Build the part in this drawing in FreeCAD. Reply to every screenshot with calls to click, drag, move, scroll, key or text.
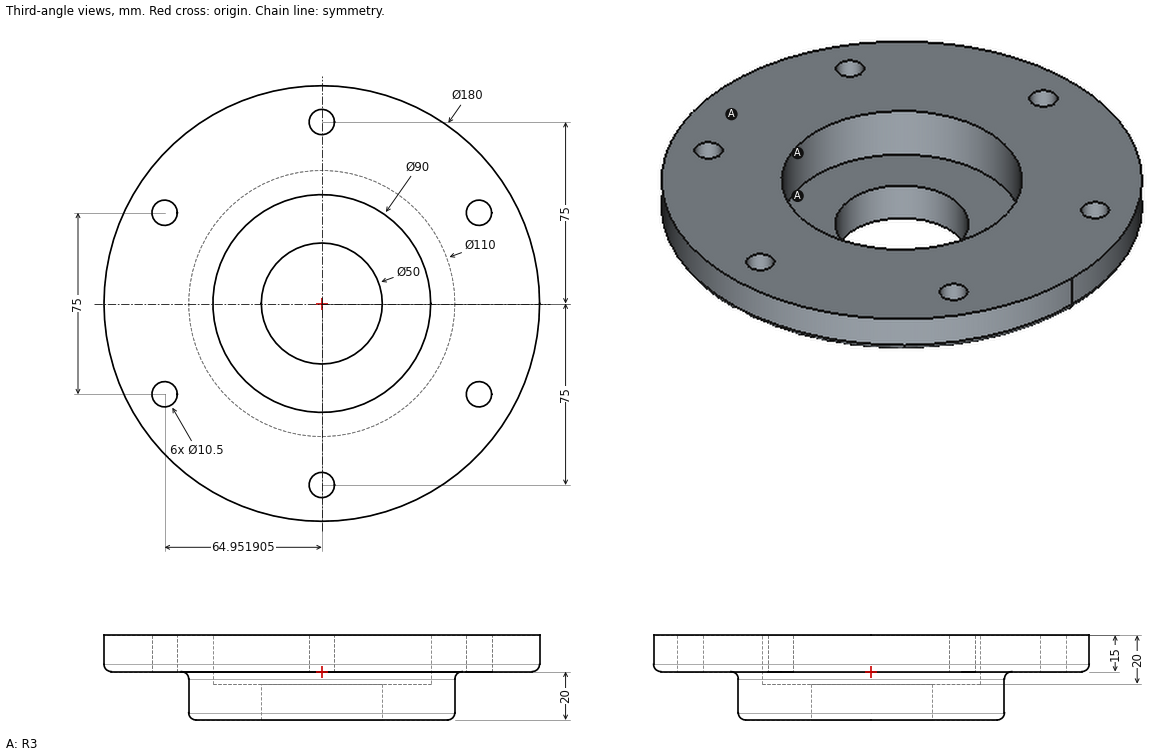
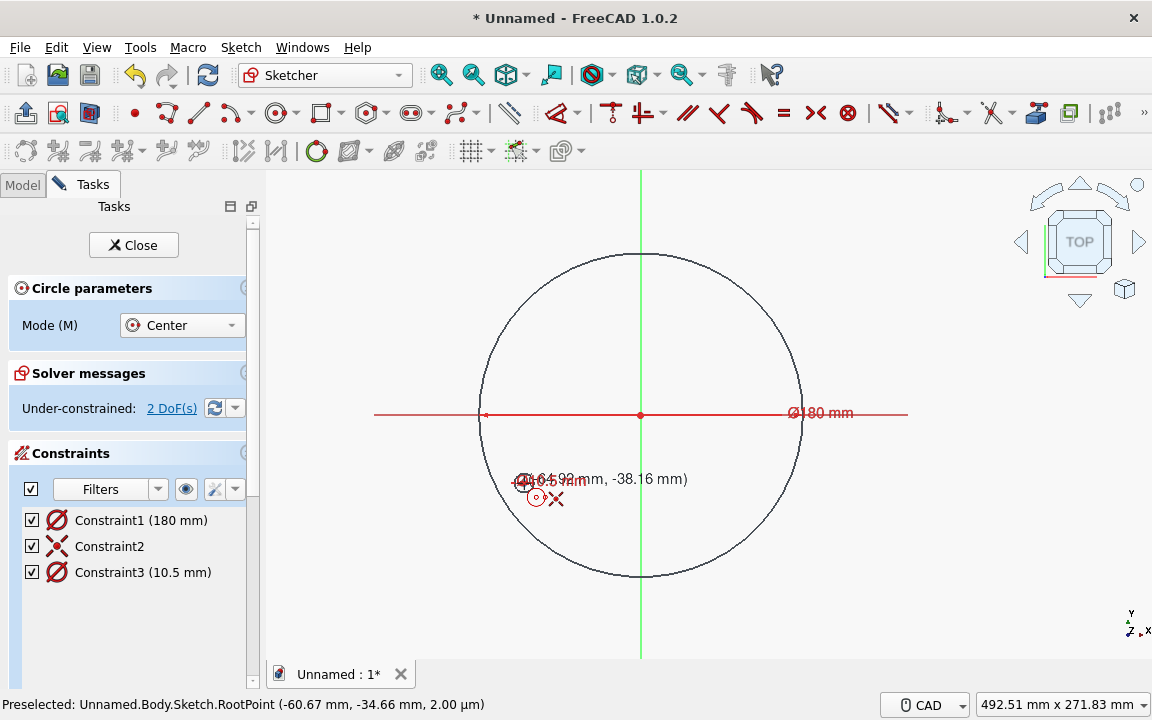
scroll(641, 550, up, 5)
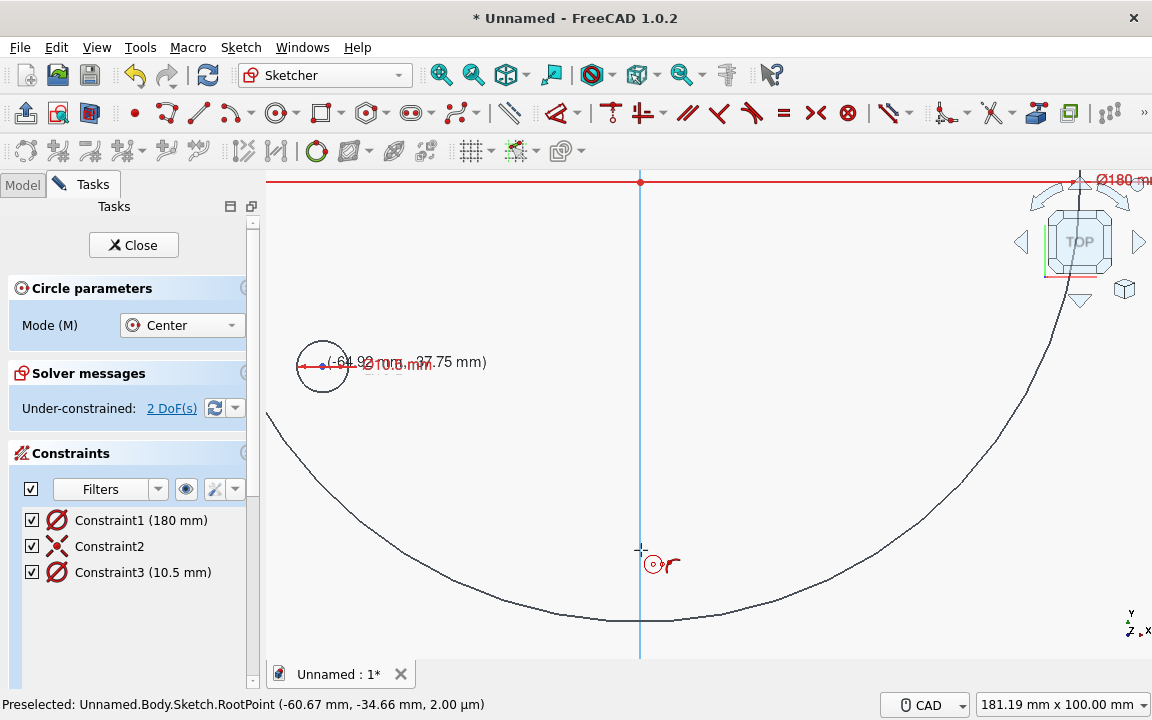
click(640, 549)
move(658, 531)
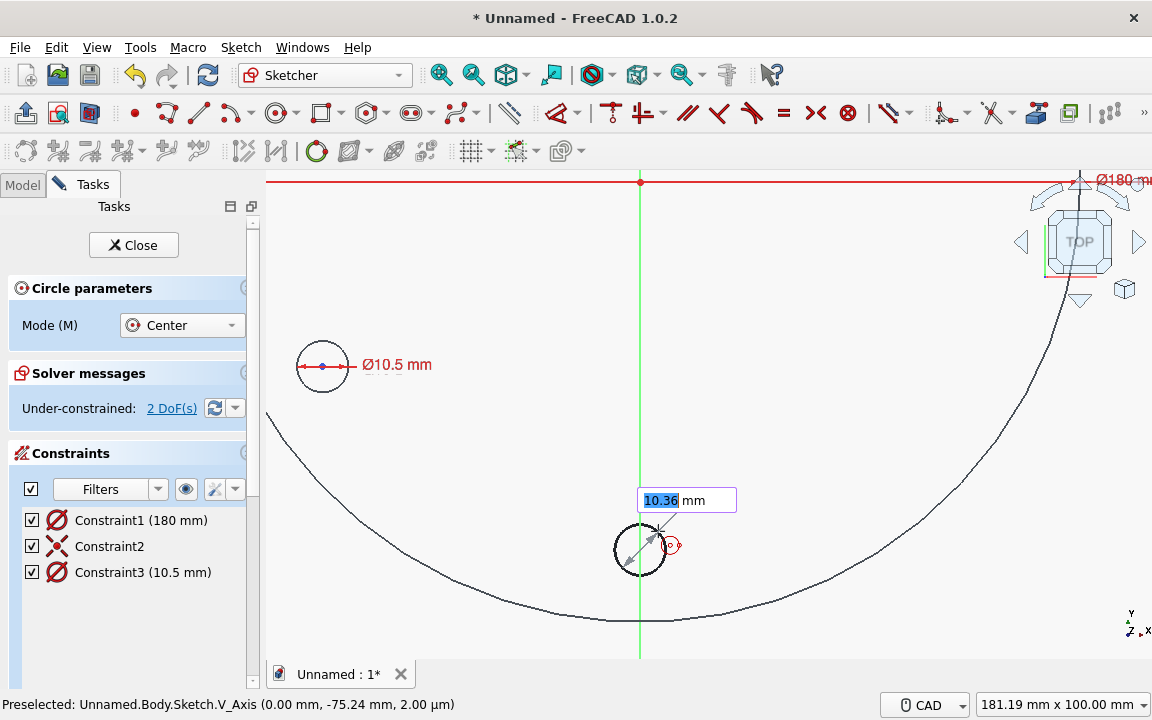
text(10.5)
key(Return)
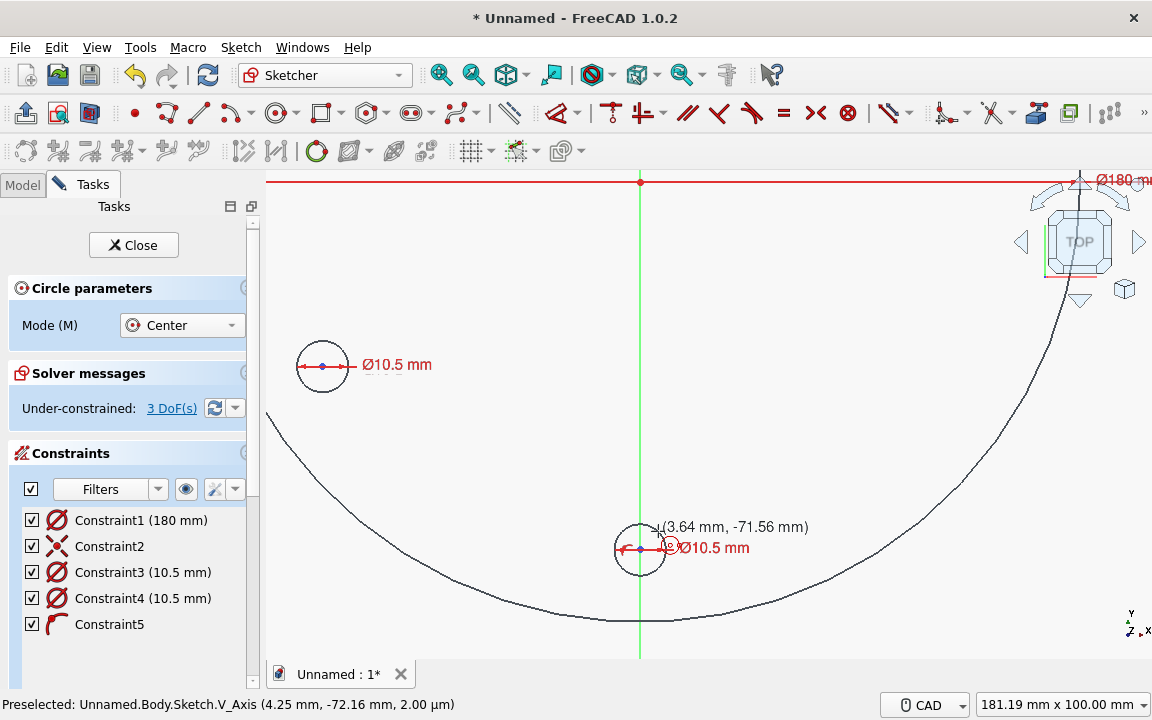
click(958, 365)
move(976, 347)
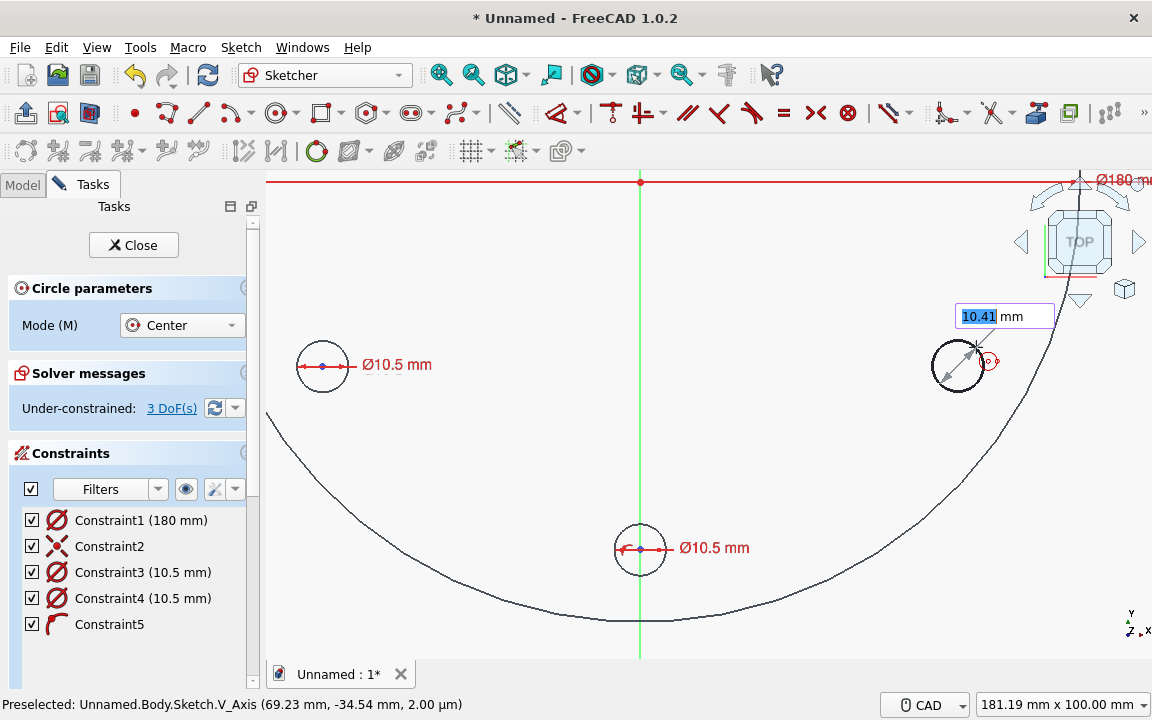
text(10.5)
key(Return)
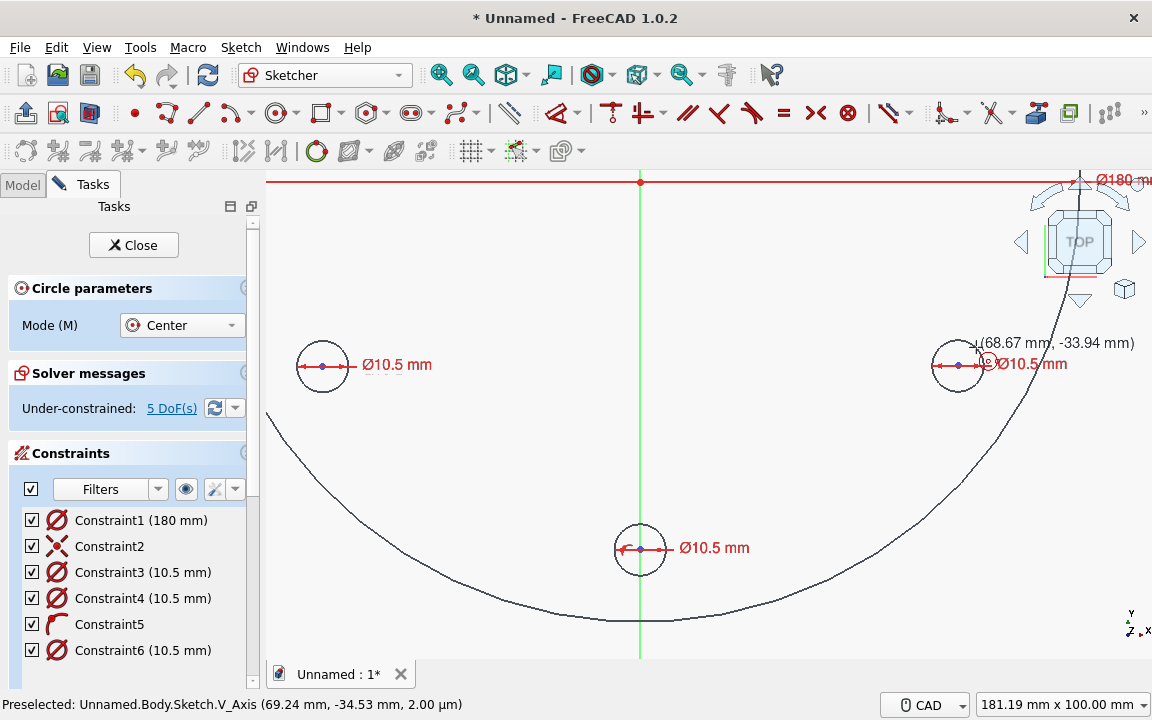
scroll(641, 550, down, 5)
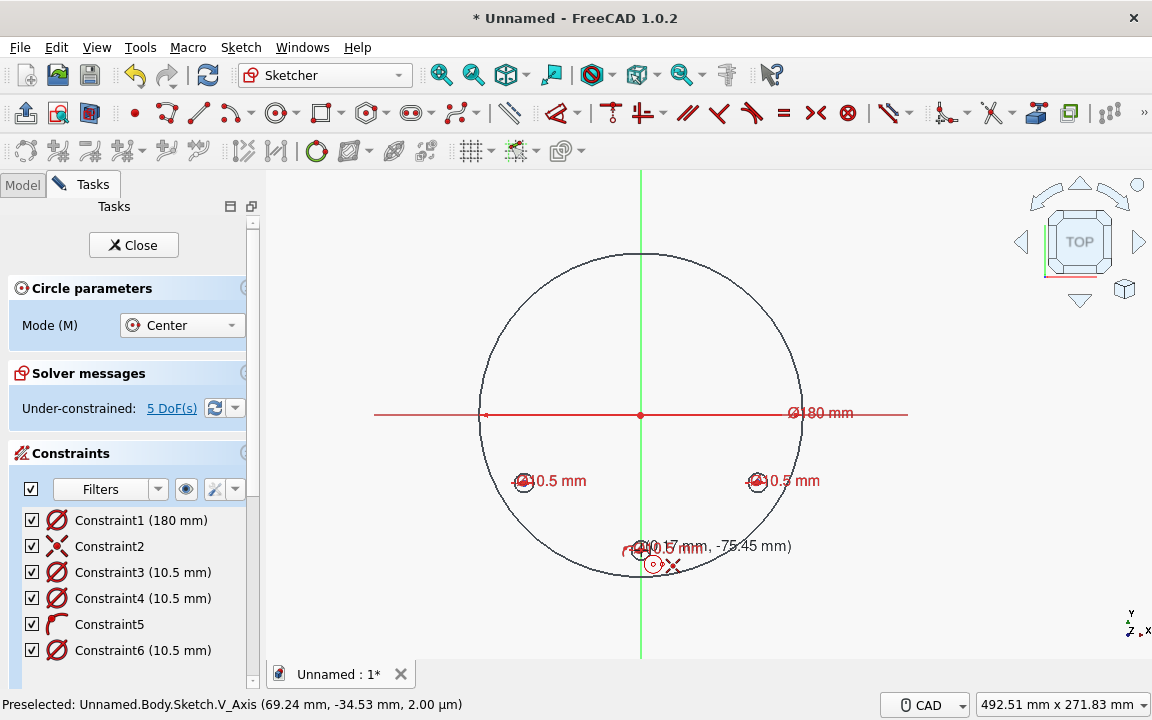
scroll(524, 348, up, 5)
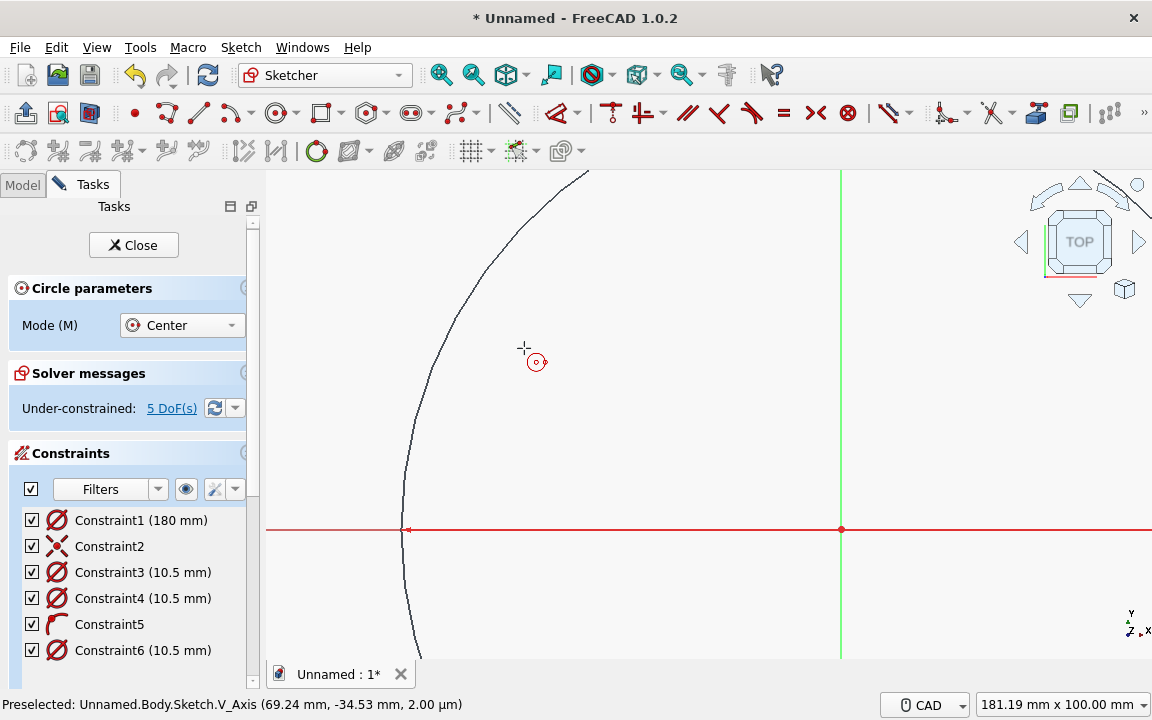
click(524, 346)
move(542, 328)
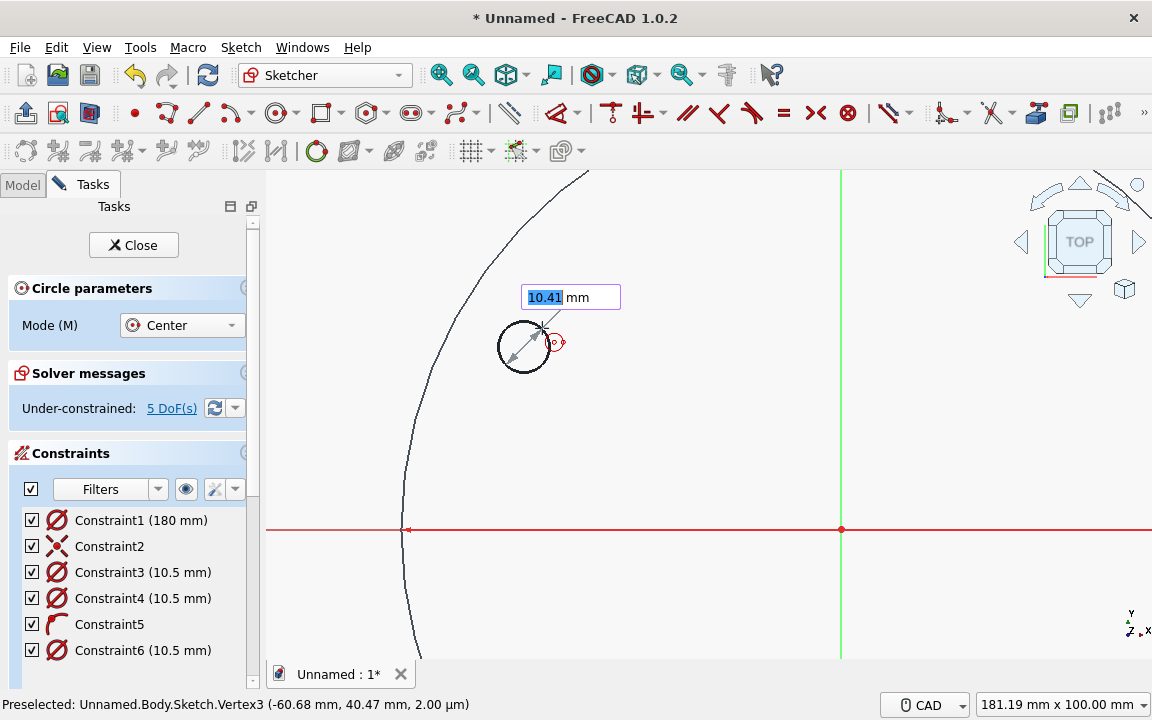
text(10.5)
key(Return)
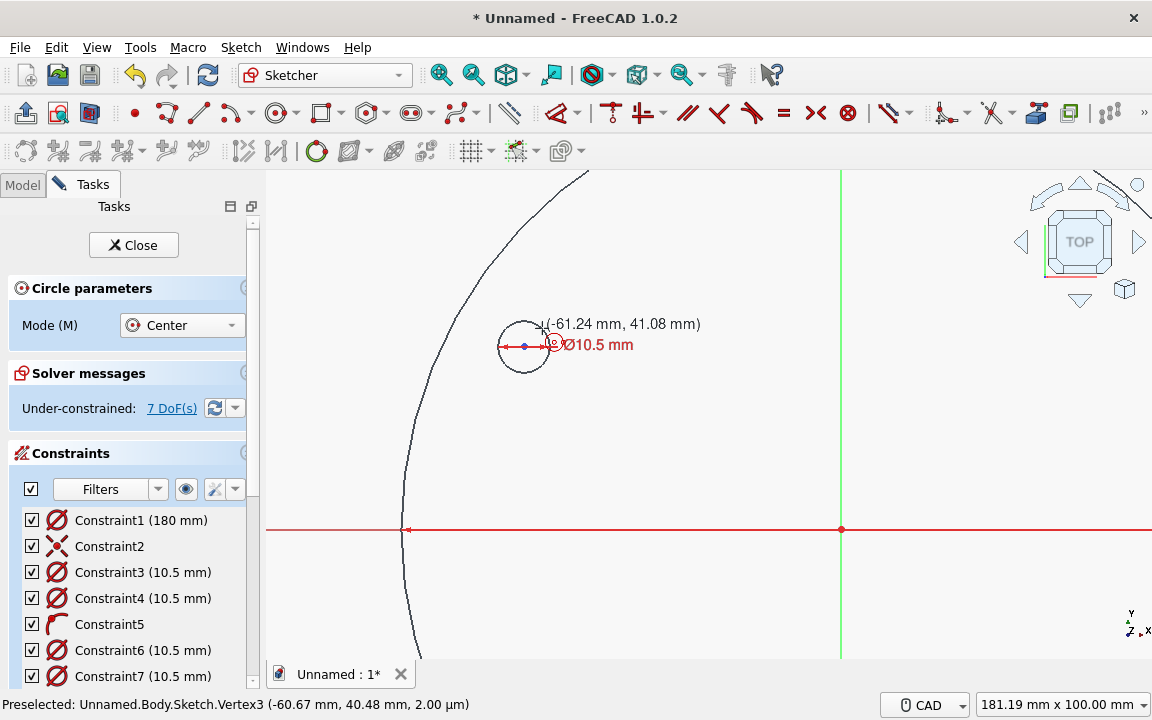
click(841, 530)
move(928, 443)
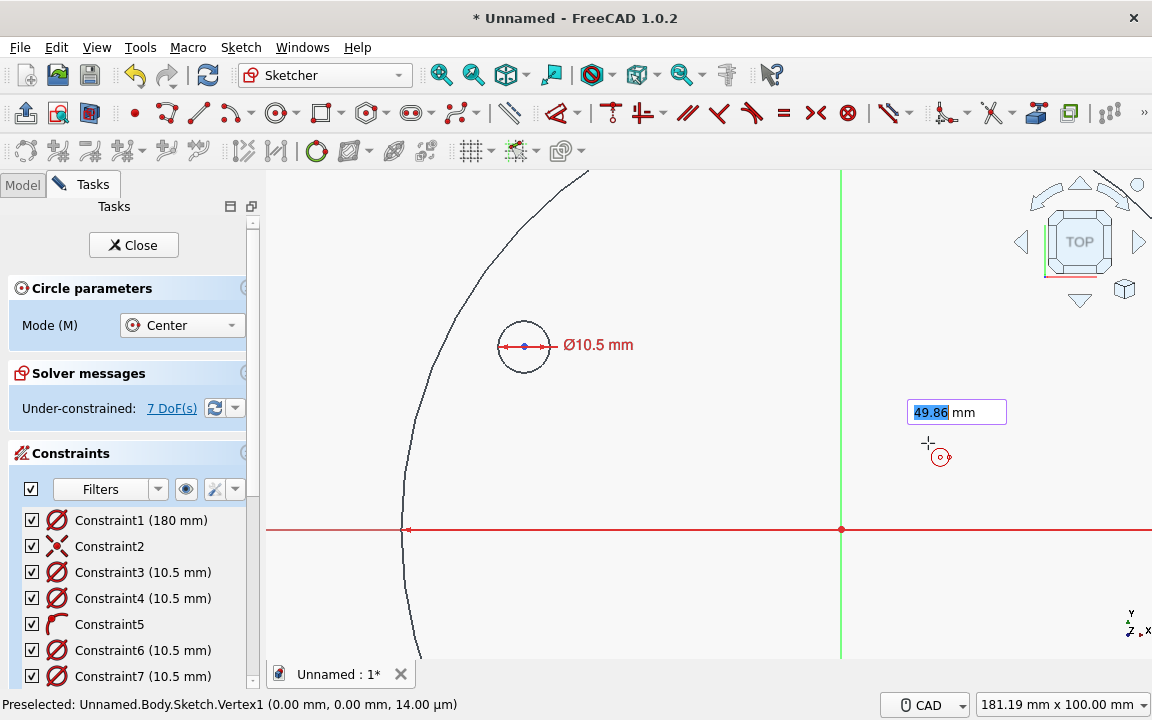
text(50)
key(Return)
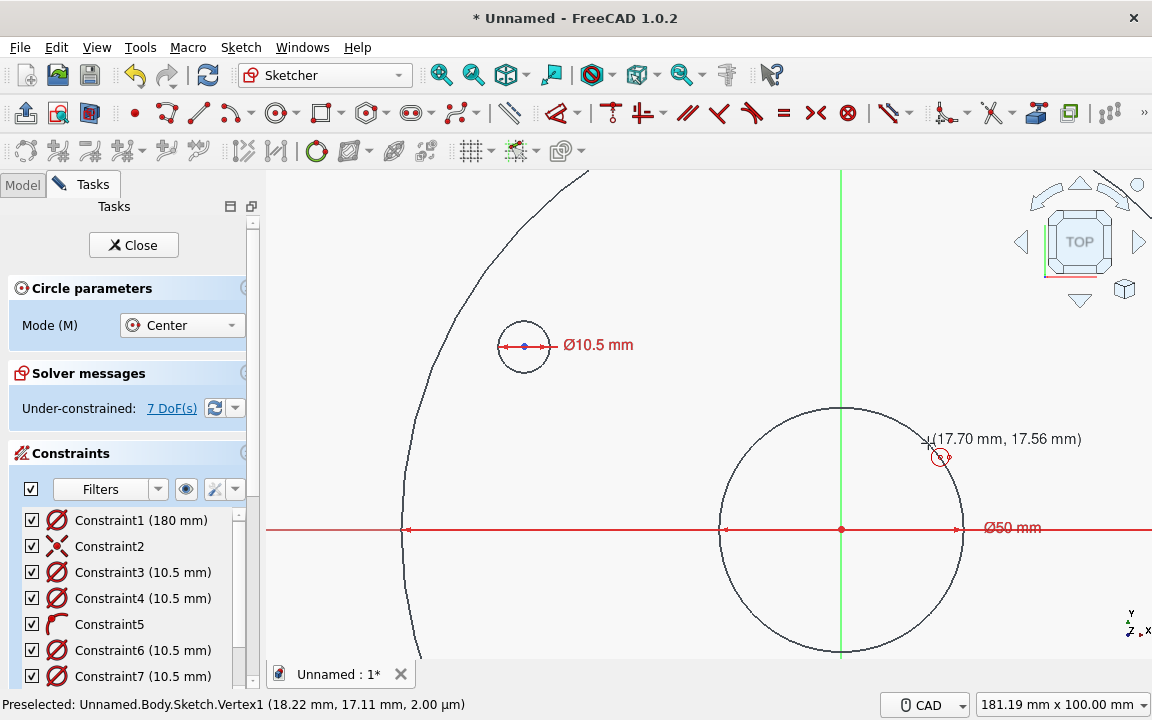
scroll(524, 347, down, 5)